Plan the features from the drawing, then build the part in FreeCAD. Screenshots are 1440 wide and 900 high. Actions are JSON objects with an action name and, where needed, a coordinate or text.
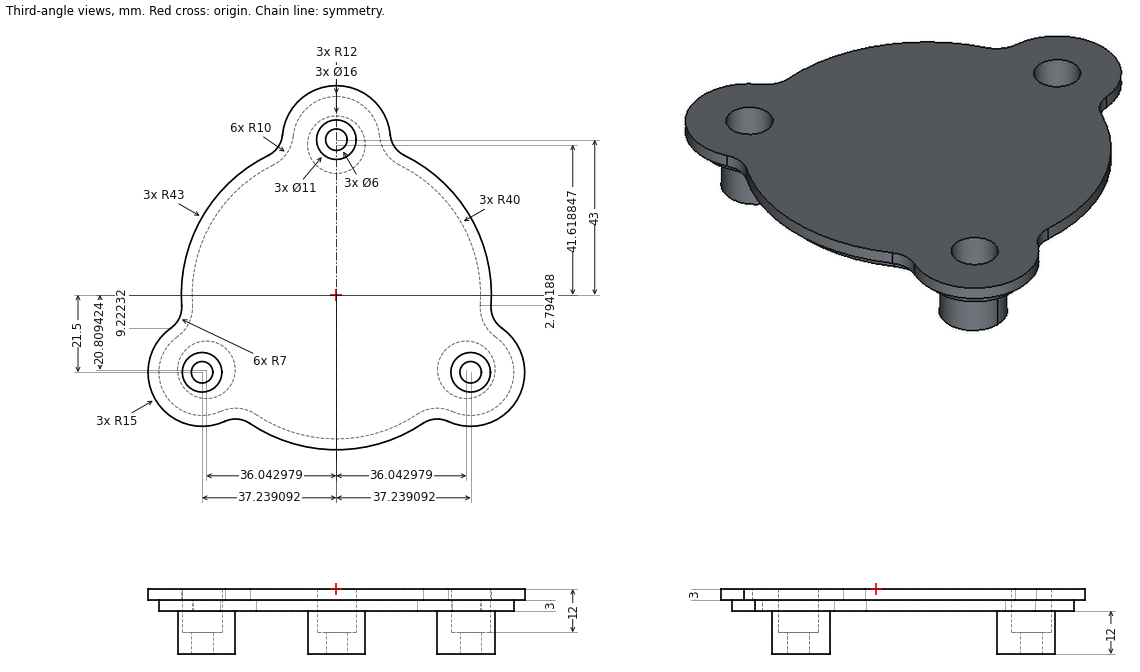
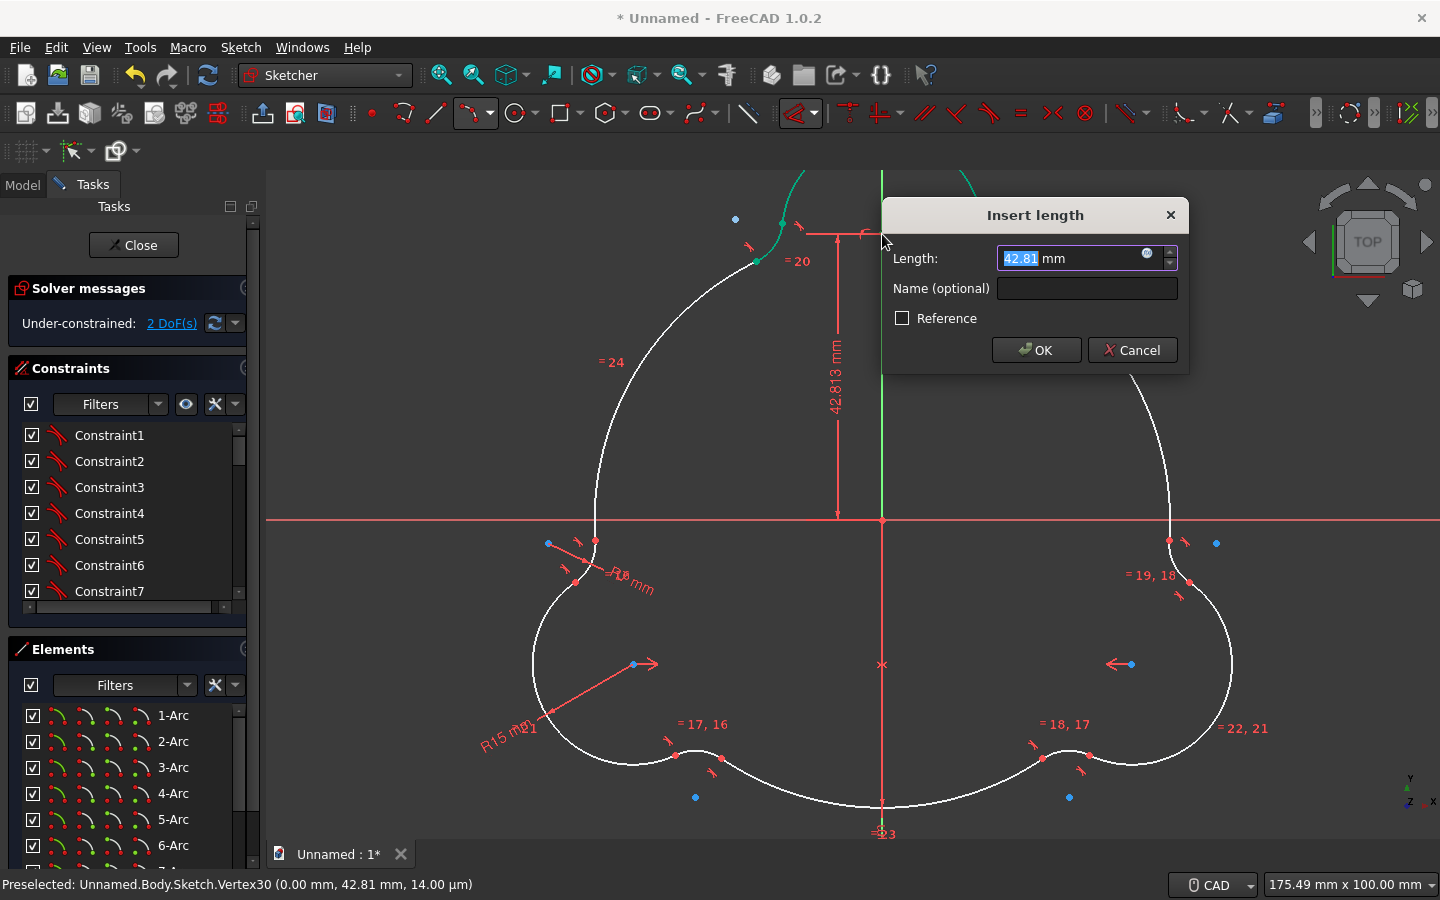
{"action": "type", "text": "43"}
{"action": "key", "text": "Return"}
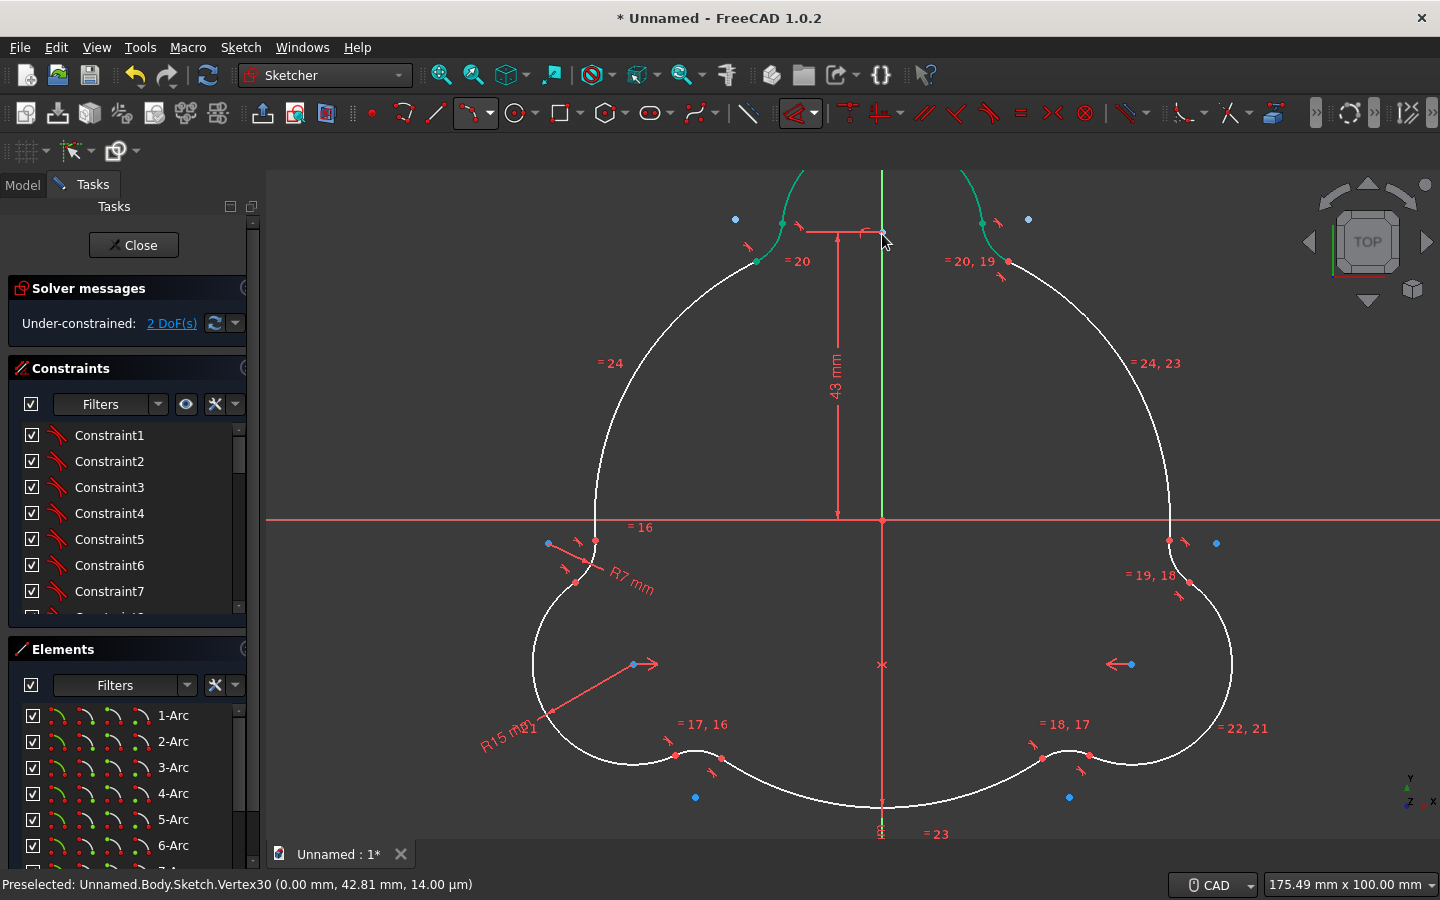
{"action": "left_click", "coordinate": [633, 664]}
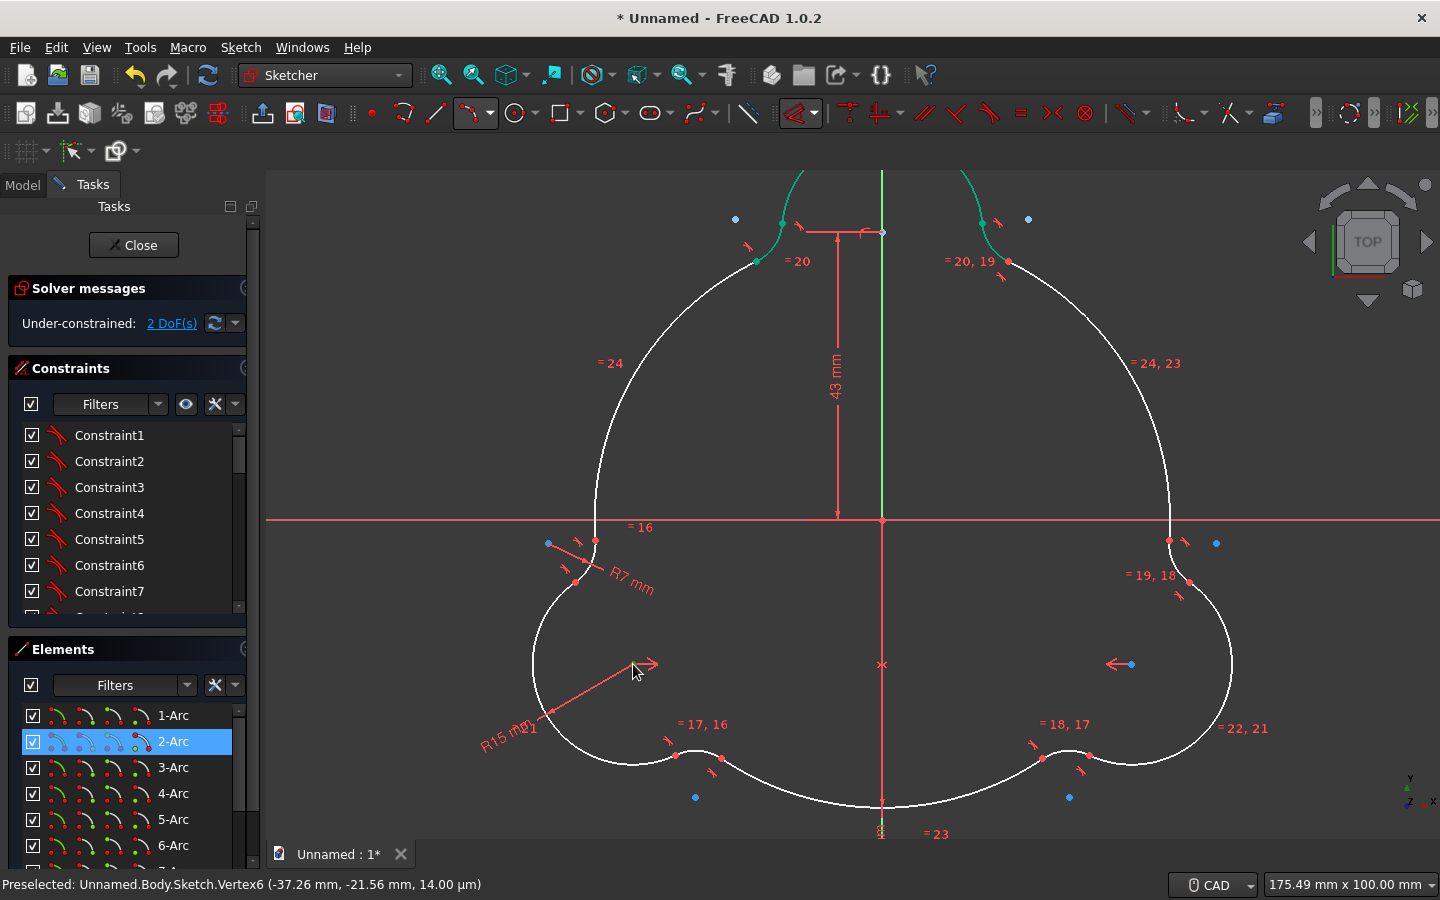
{"action": "left_click", "coordinate": [816, 114]}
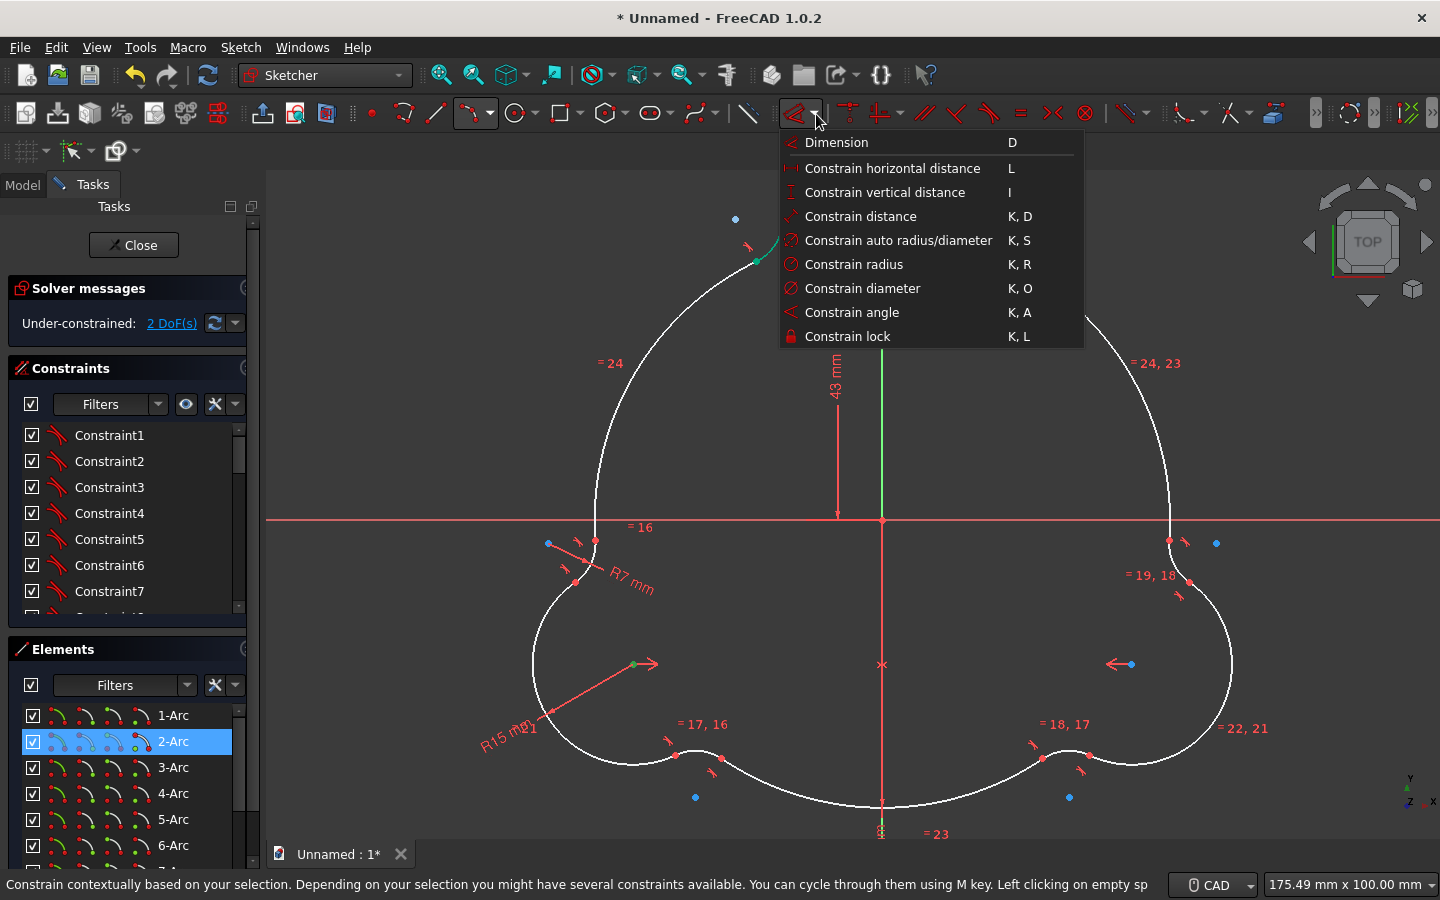
{"action": "left_click", "coordinate": [932, 192]}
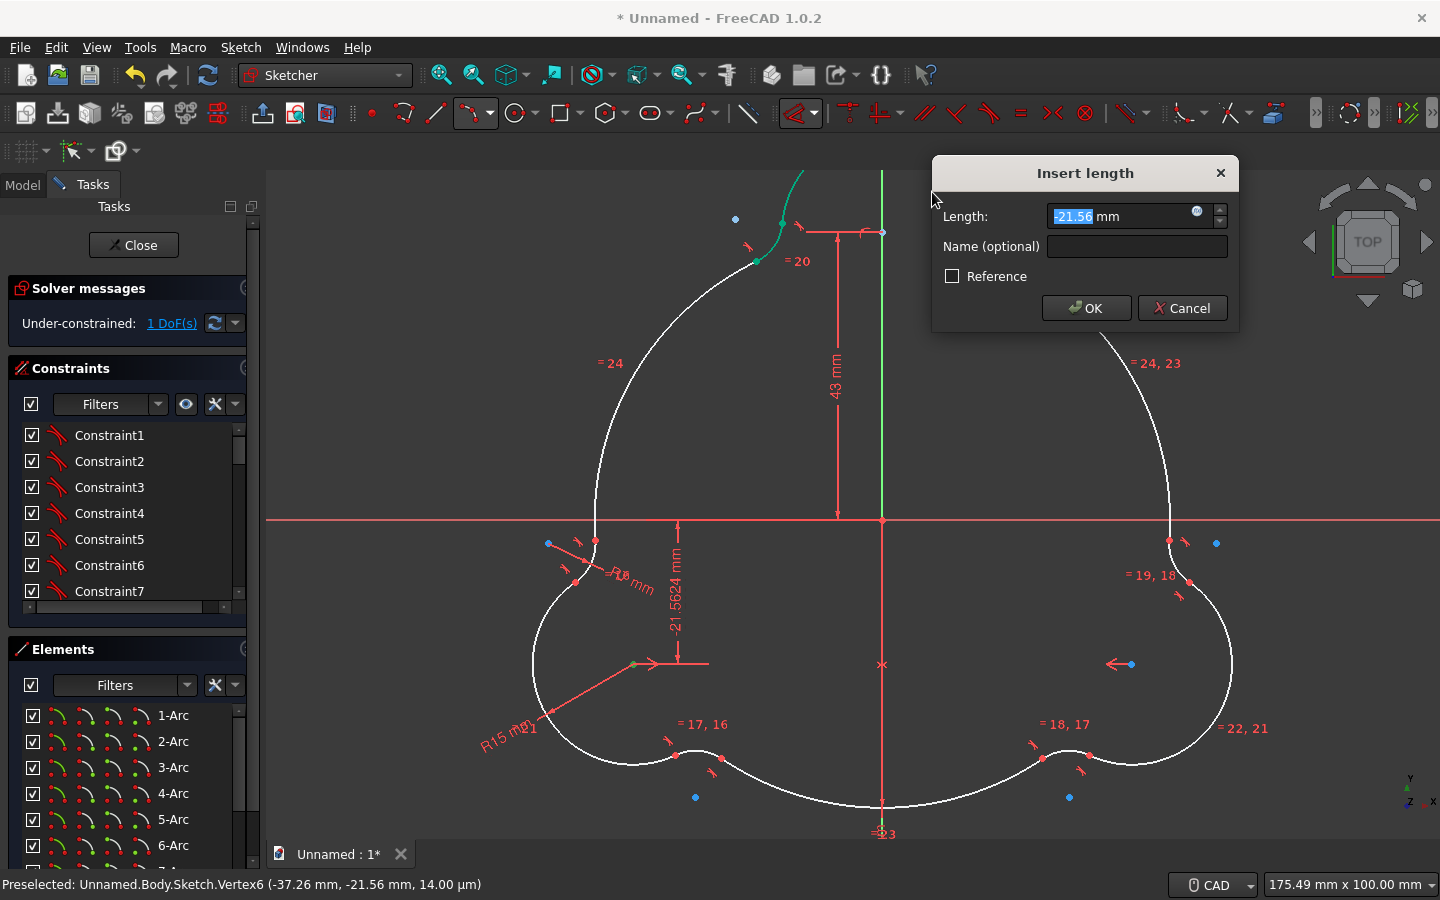
{"action": "type", "text": "-21.5"}
{"action": "key", "text": "Return"}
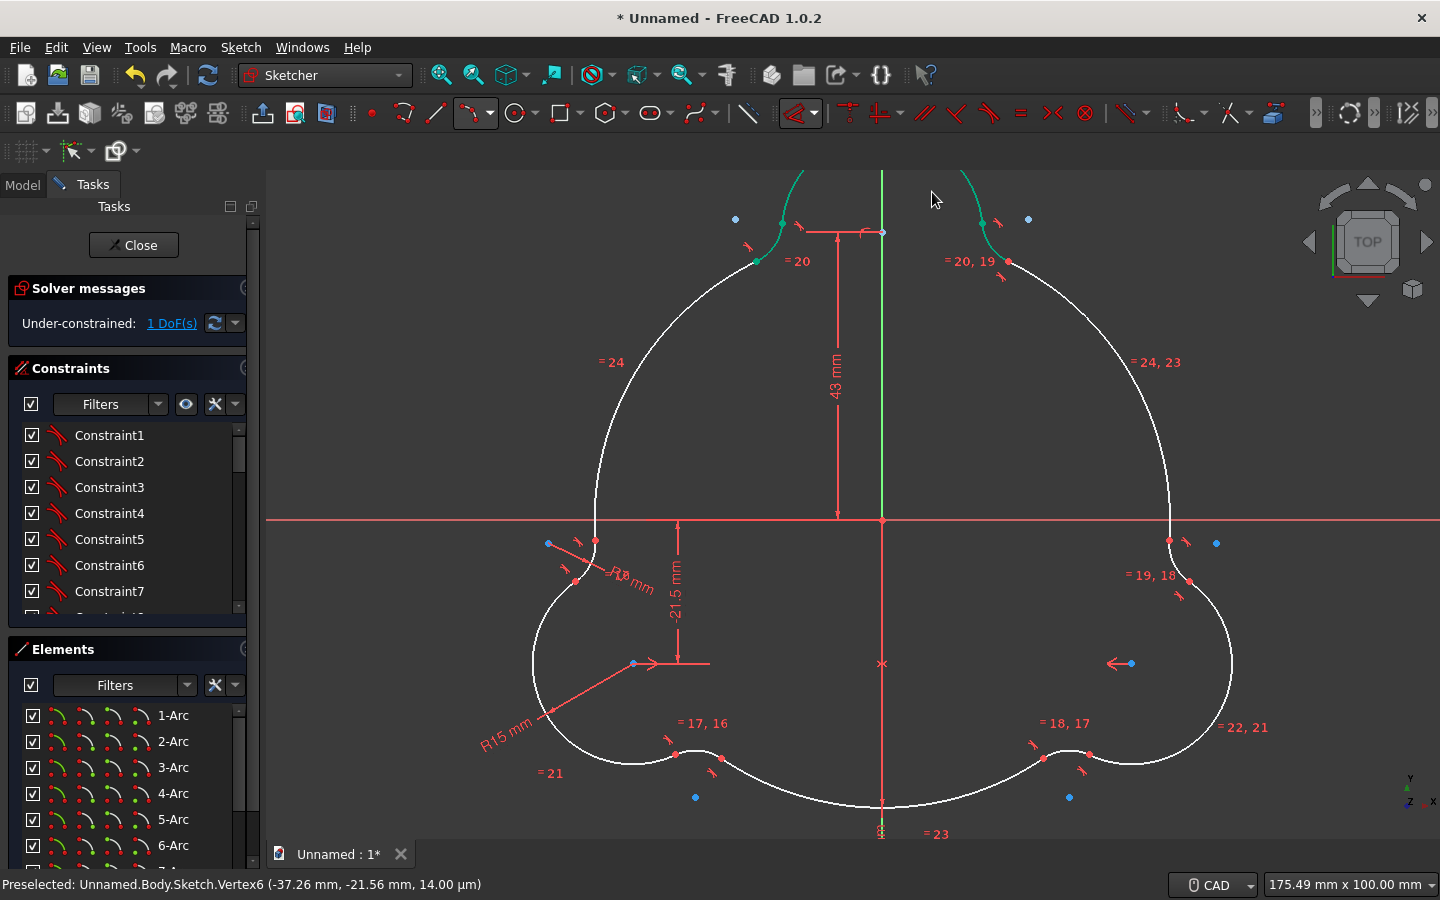
{"action": "left_click", "coordinate": [576, 582]}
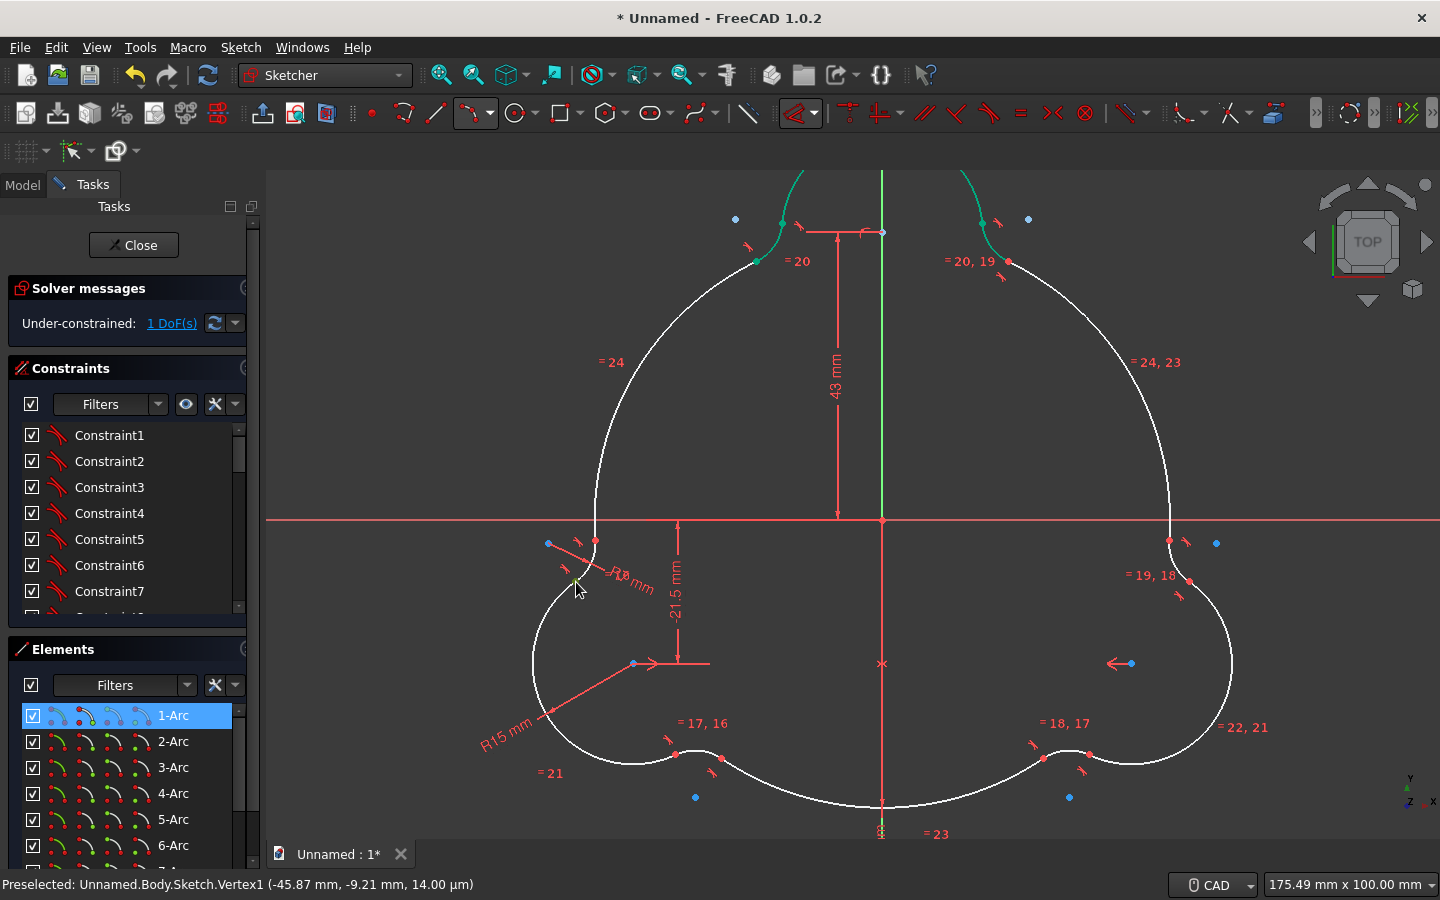
{"action": "left_click", "coordinate": [816, 114]}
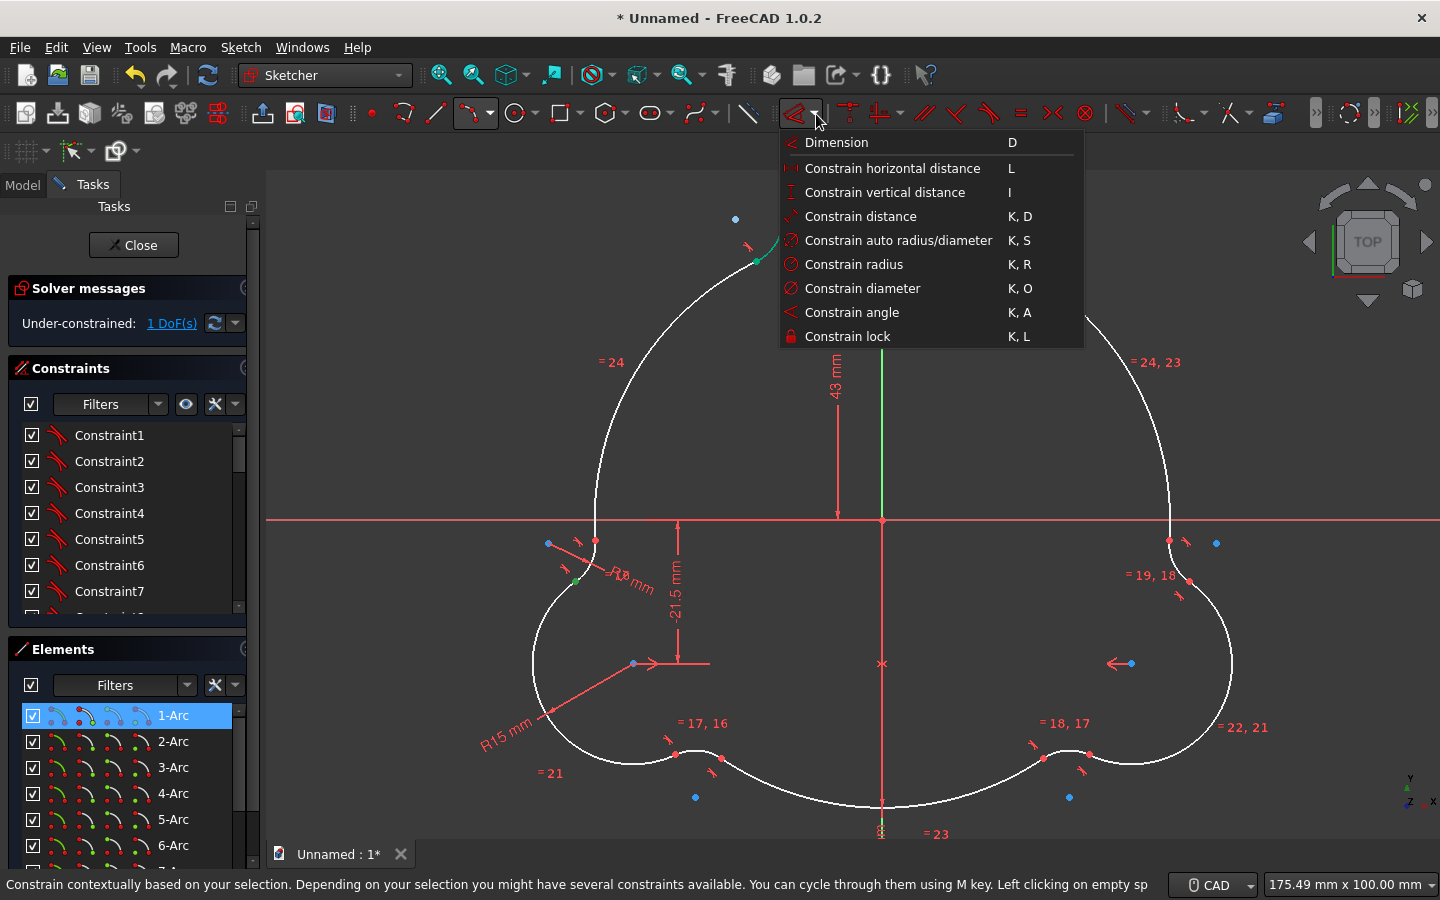
{"action": "left_click", "coordinate": [932, 192]}